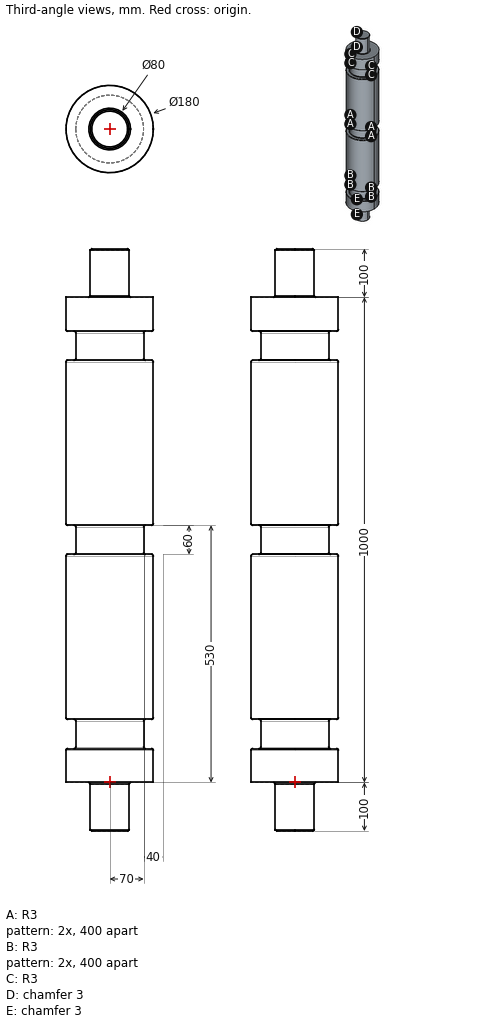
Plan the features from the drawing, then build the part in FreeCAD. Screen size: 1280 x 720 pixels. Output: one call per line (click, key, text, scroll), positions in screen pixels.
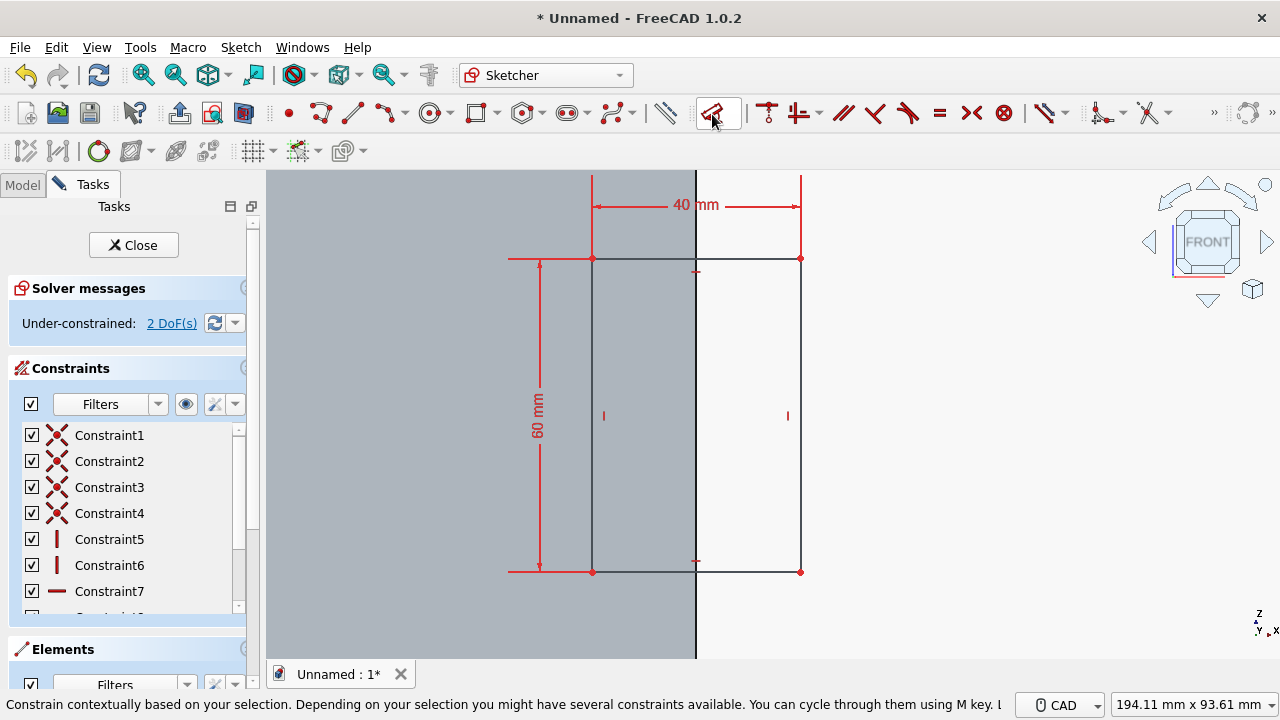
click(592, 259)
click(443, 225)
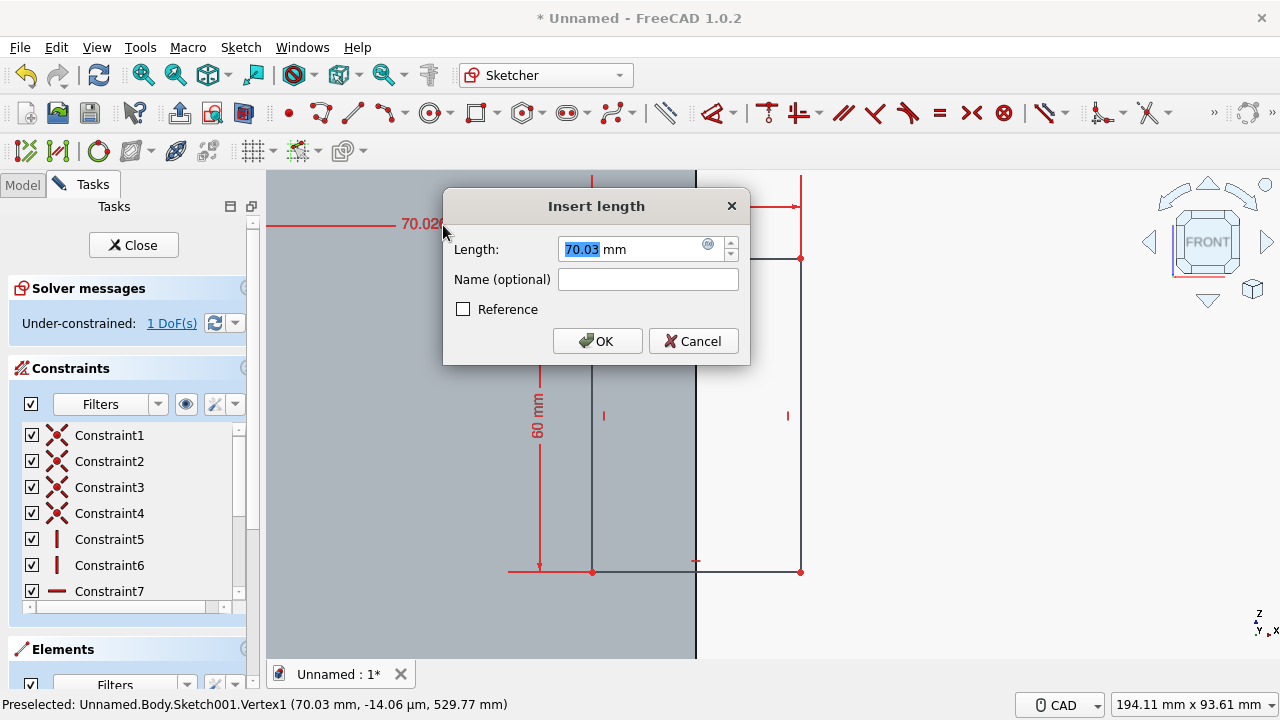
text(70)
key(Return)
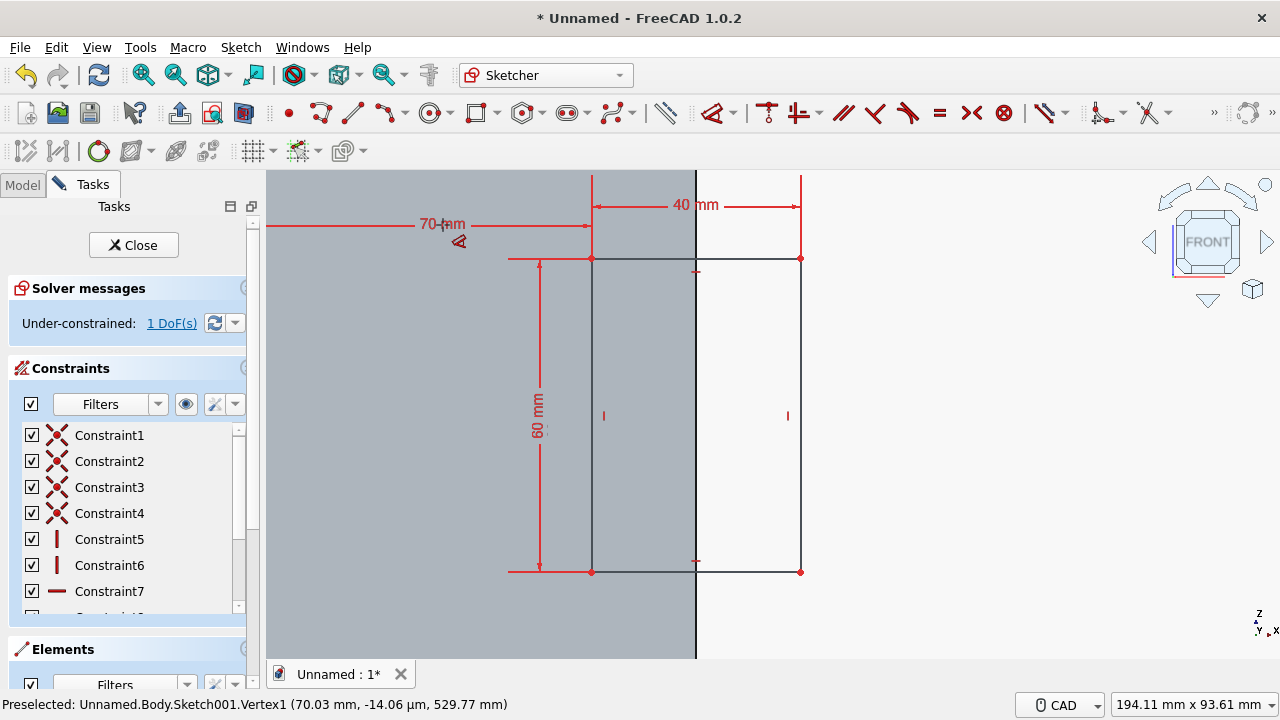
click(592, 259)
click(626, 445)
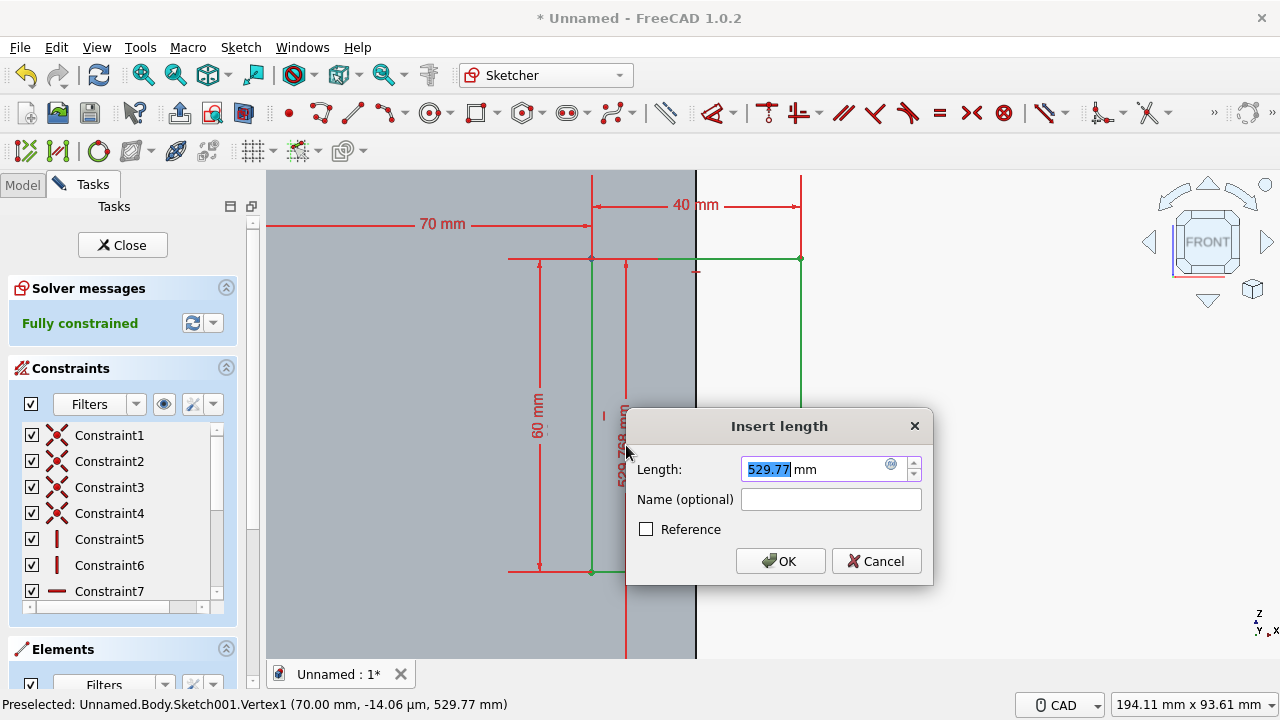
text(530)
key(Return)
key(Escape)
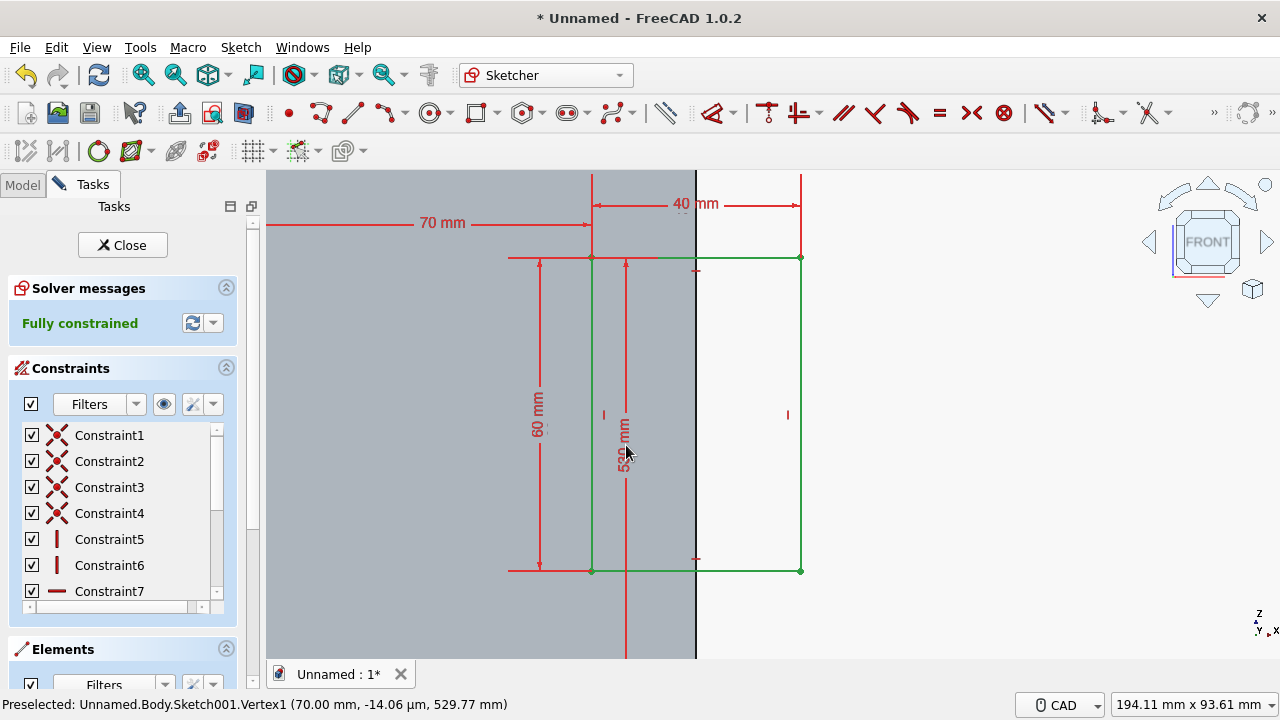
click(123, 245)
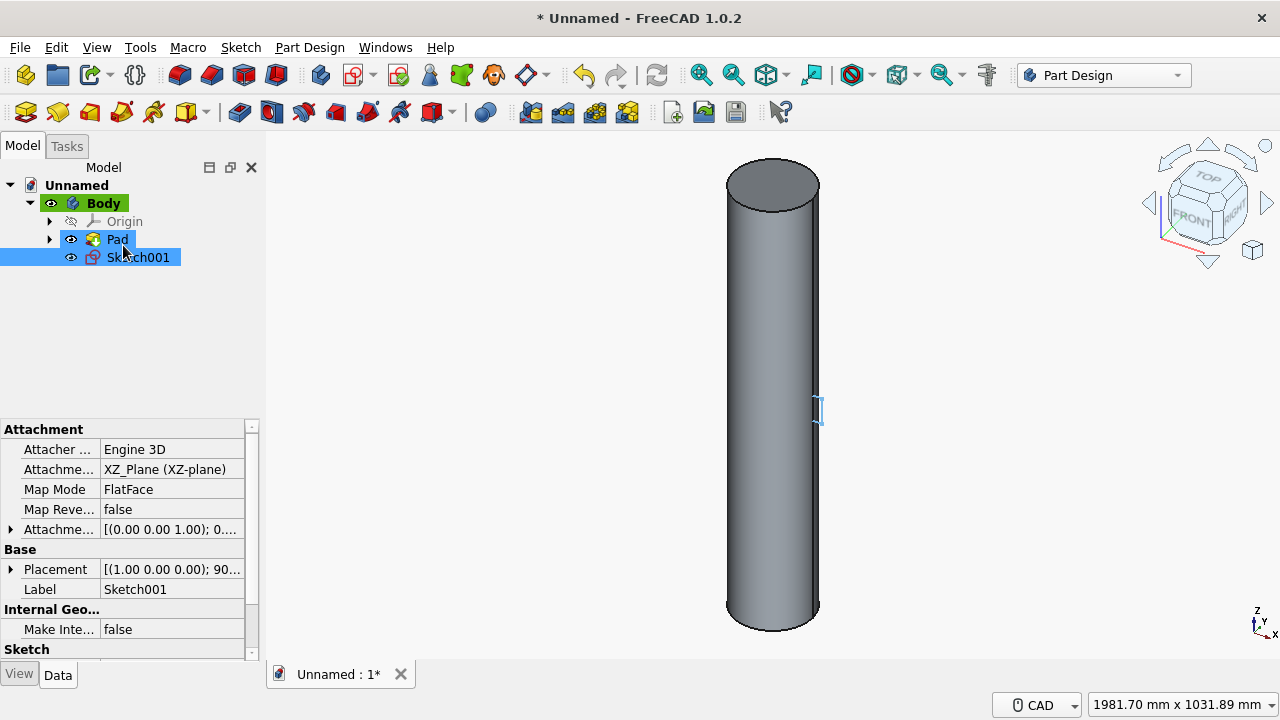
click(304, 112)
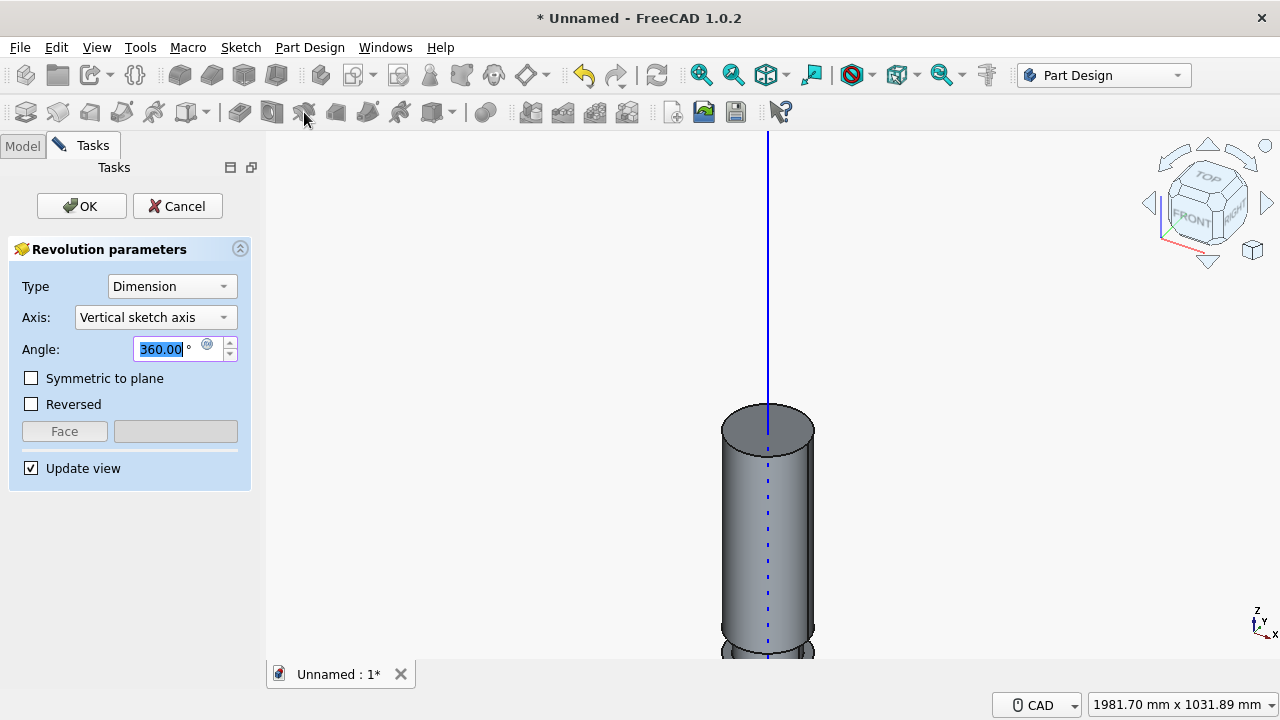
click(82, 206)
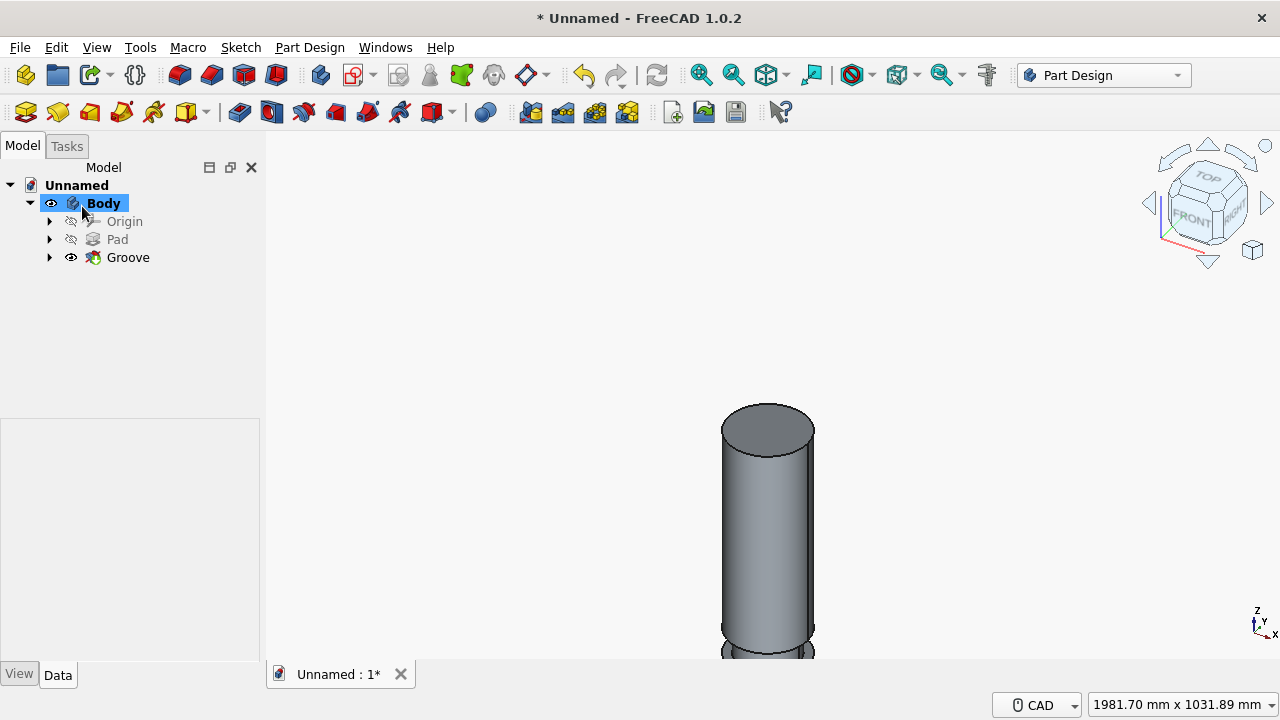
click(702, 76)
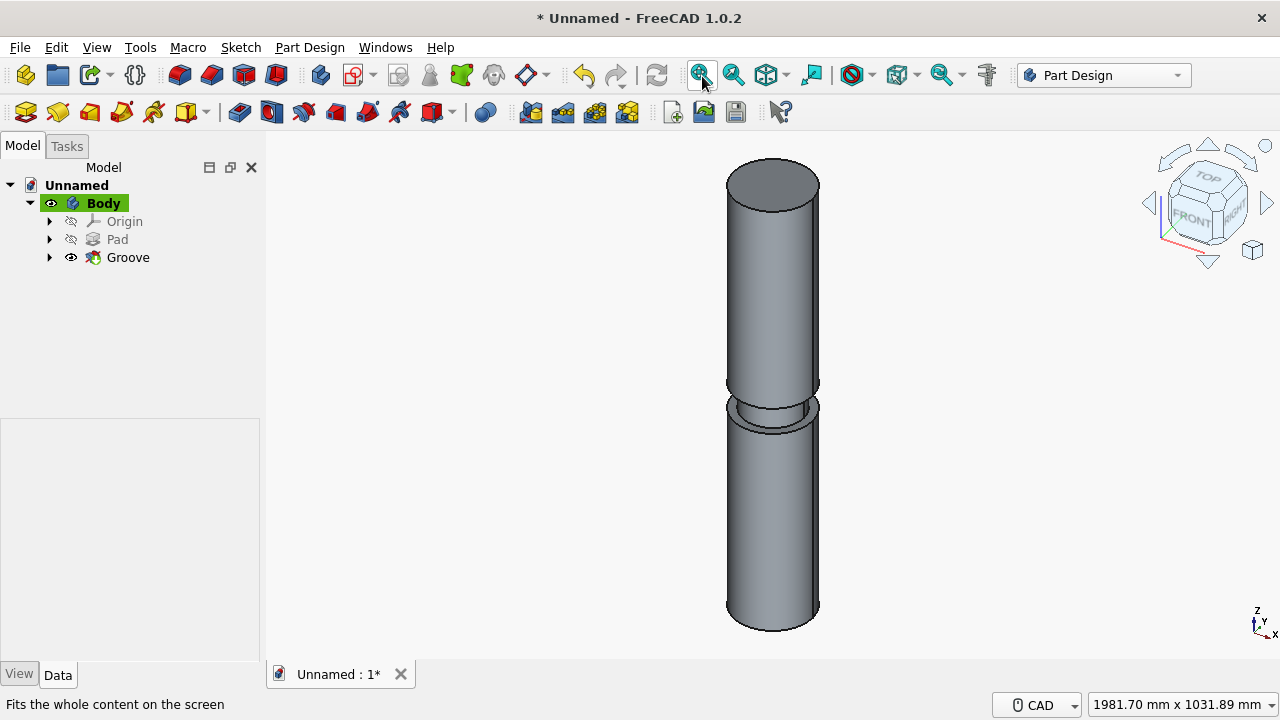
click(727, 409)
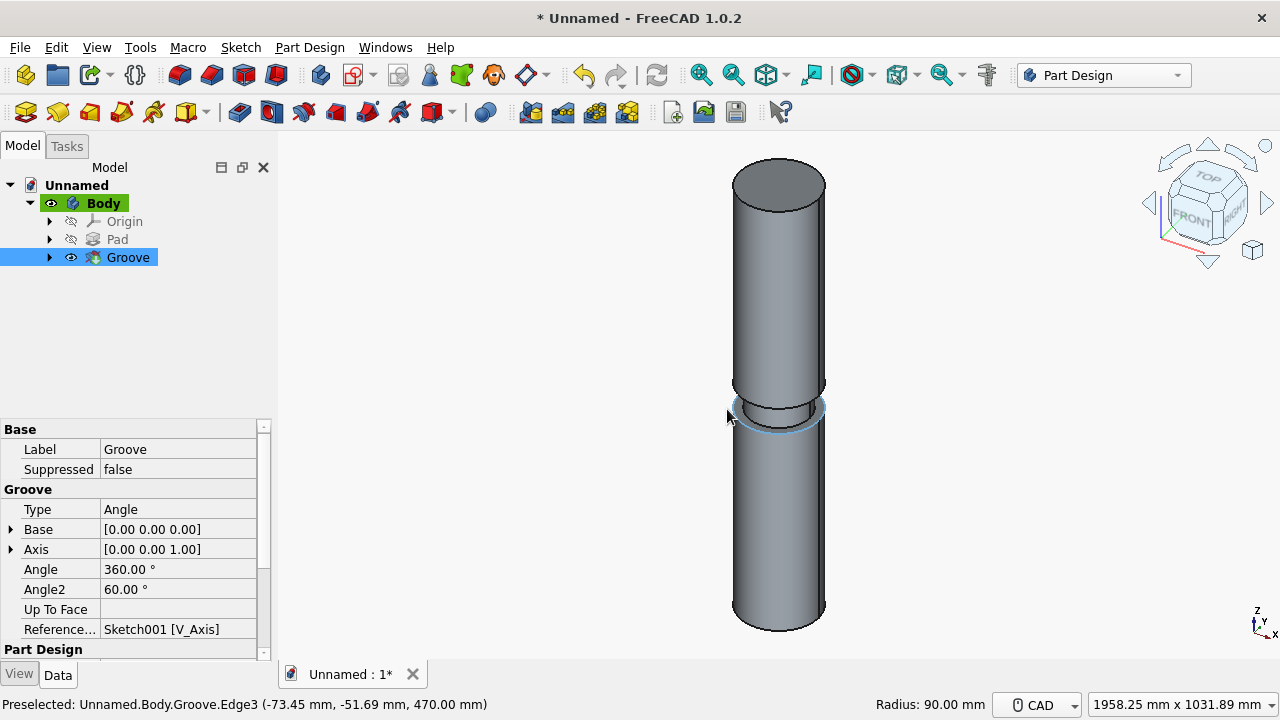
key(0)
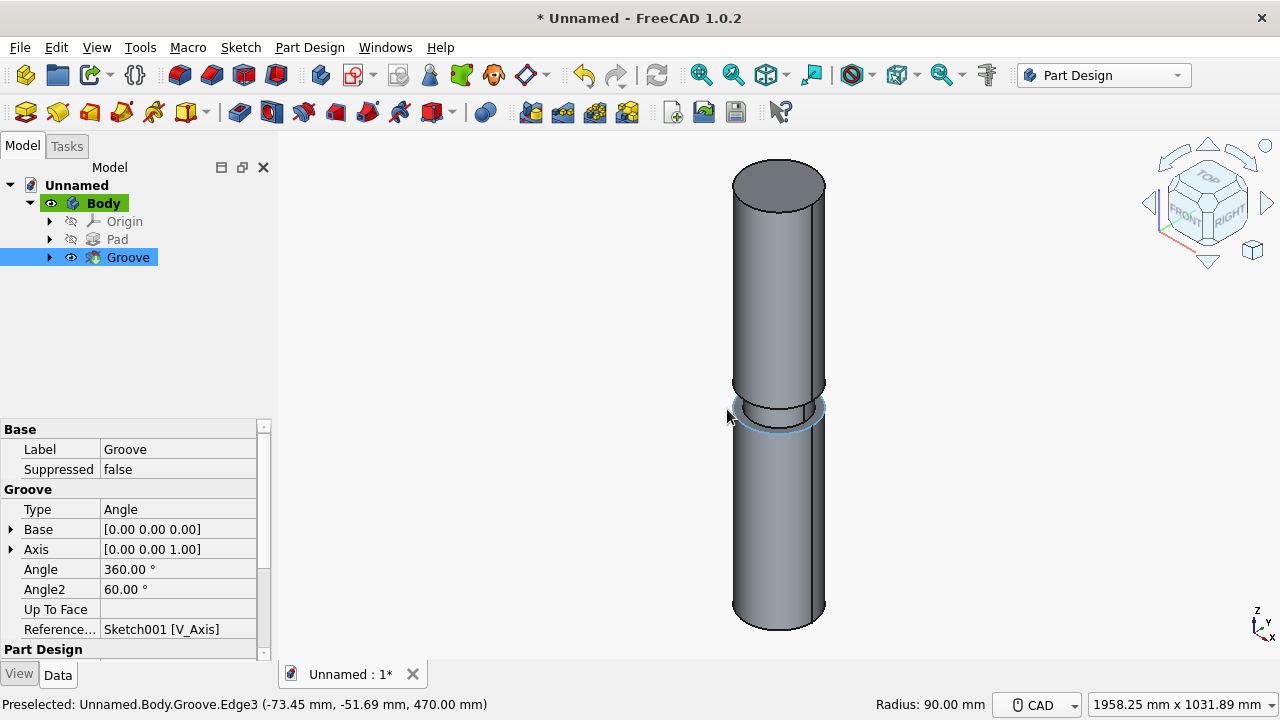
click(738, 394, ctrl)